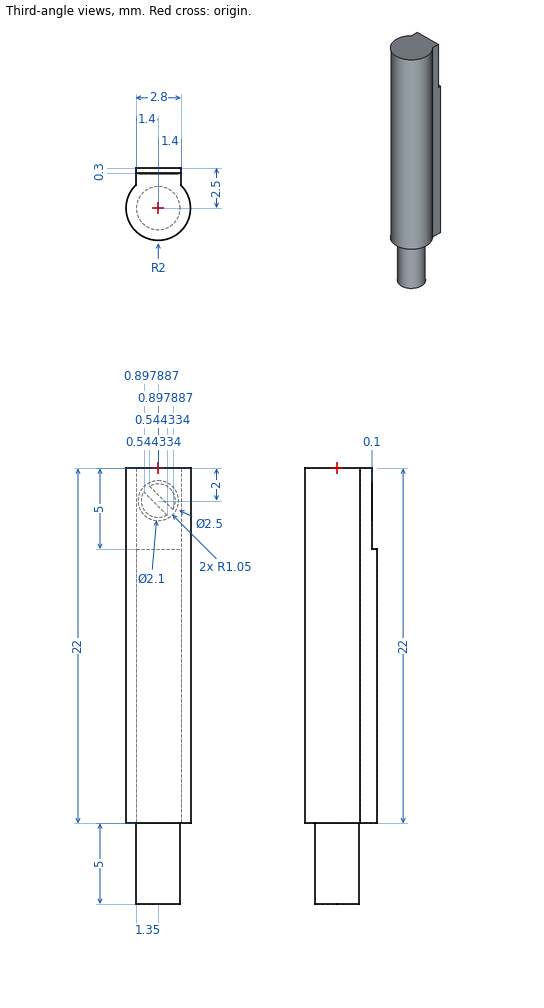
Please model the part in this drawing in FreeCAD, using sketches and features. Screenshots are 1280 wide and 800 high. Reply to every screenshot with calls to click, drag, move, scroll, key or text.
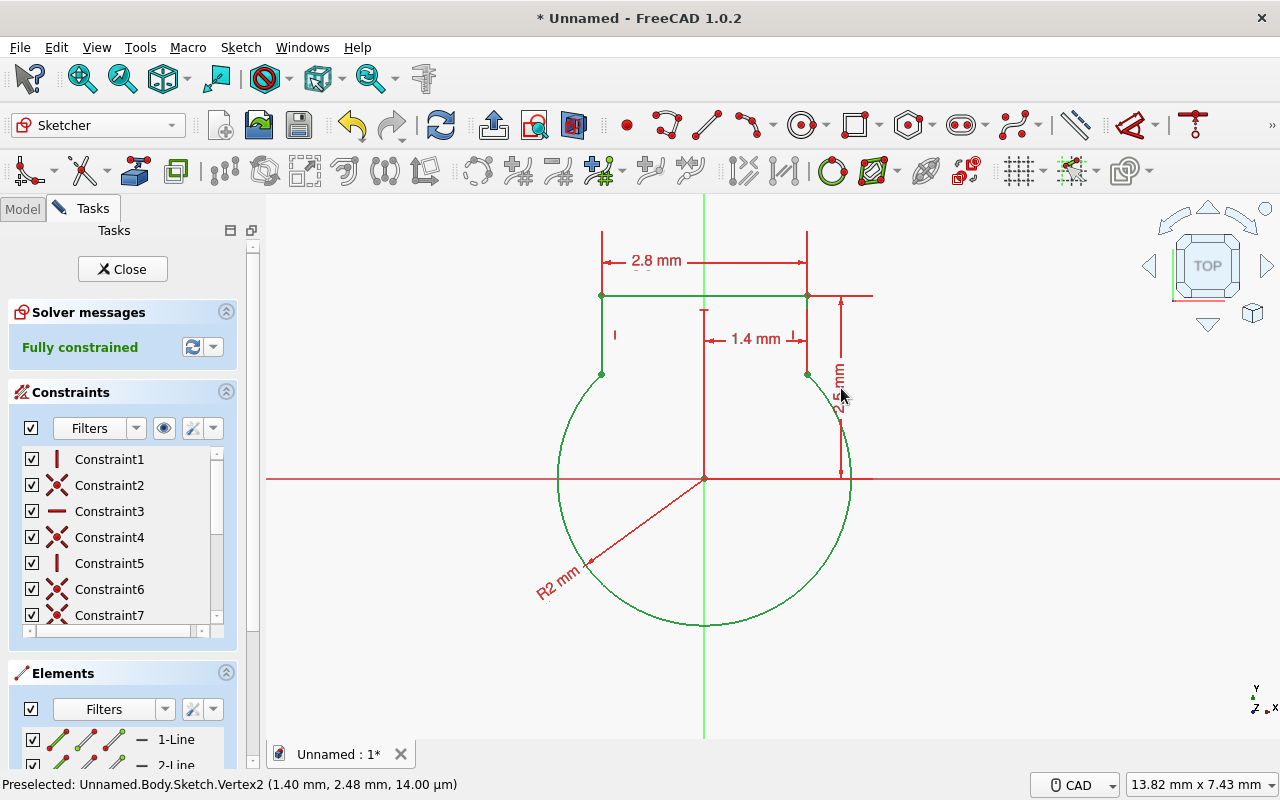
click(123, 269)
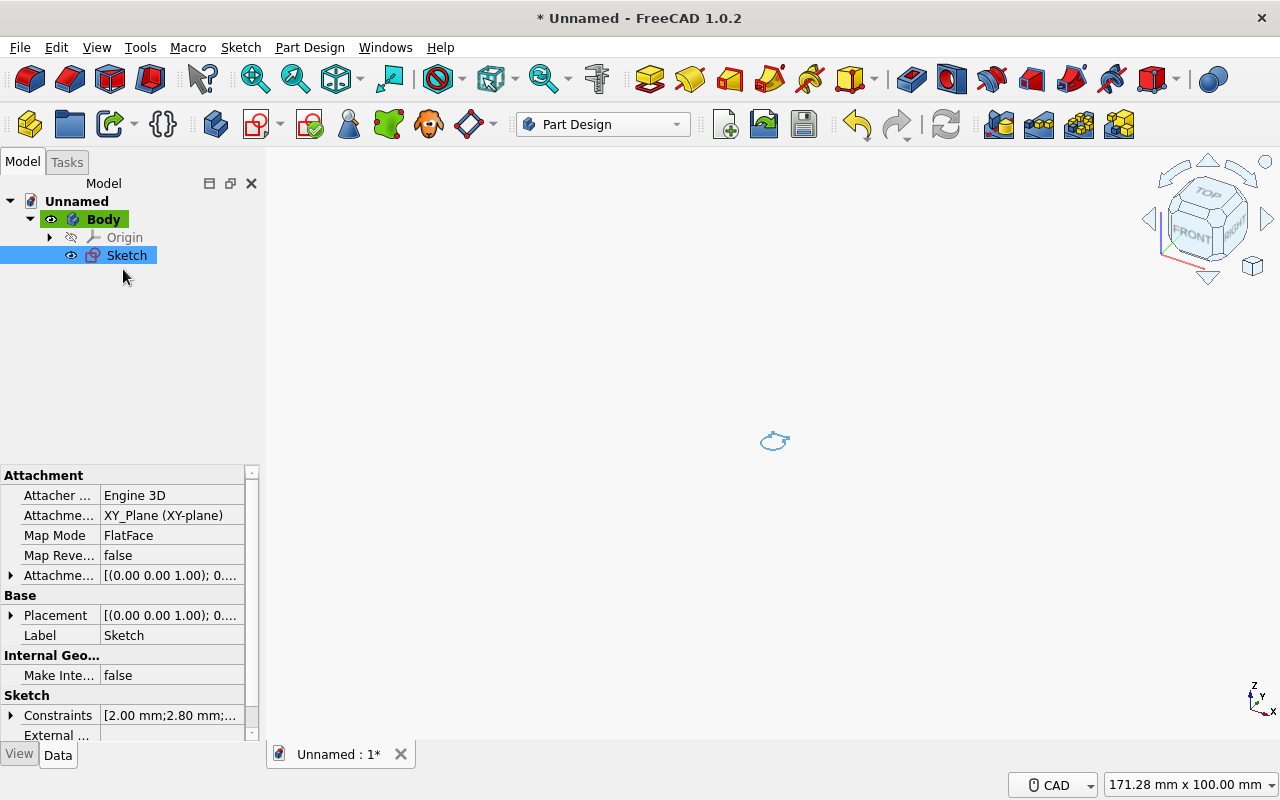
click(650, 80)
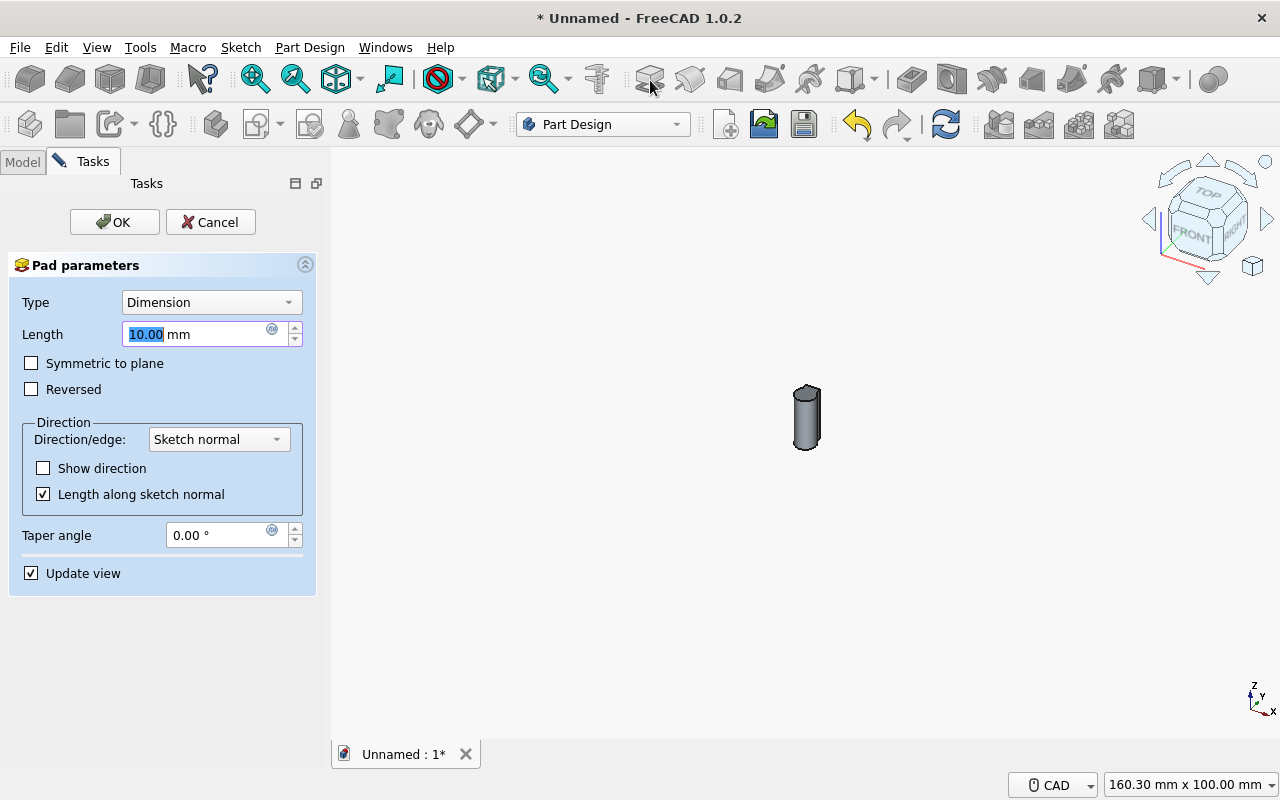
text(22)
key(Tab)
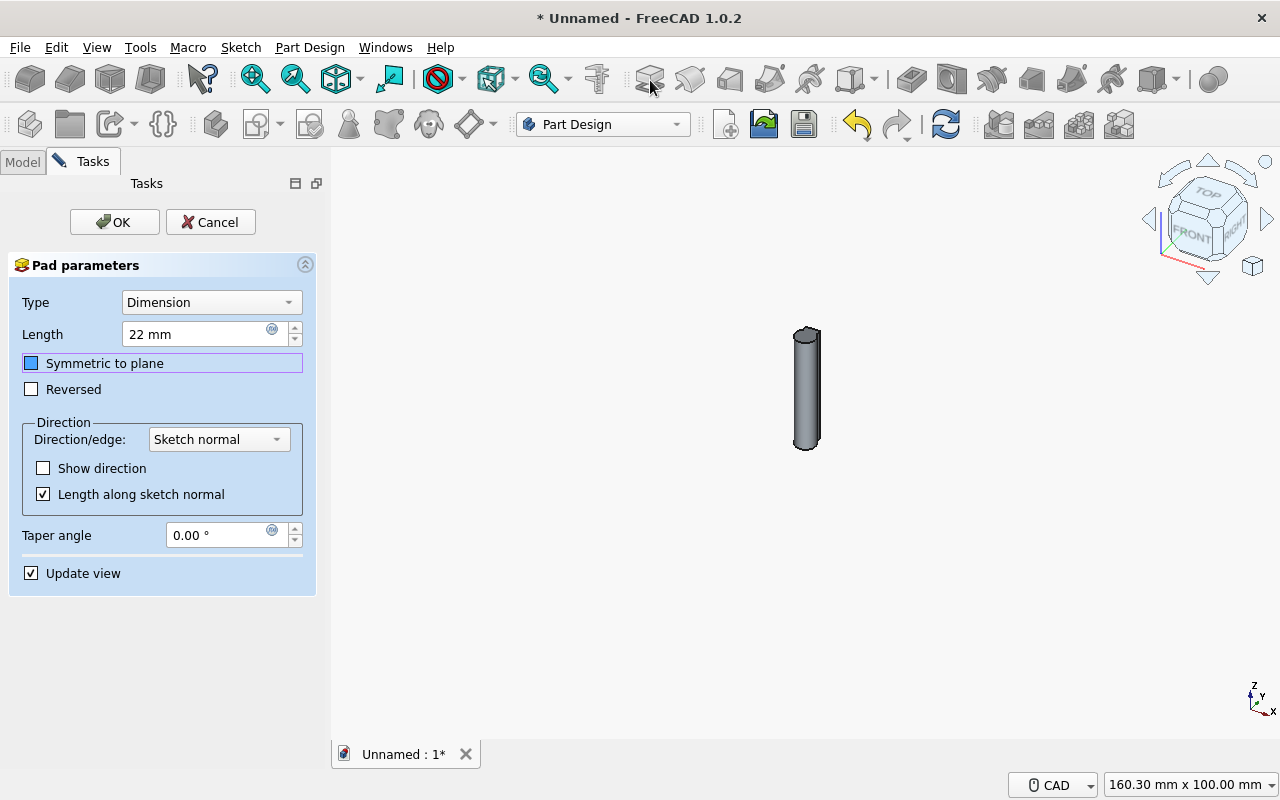
click(30, 389)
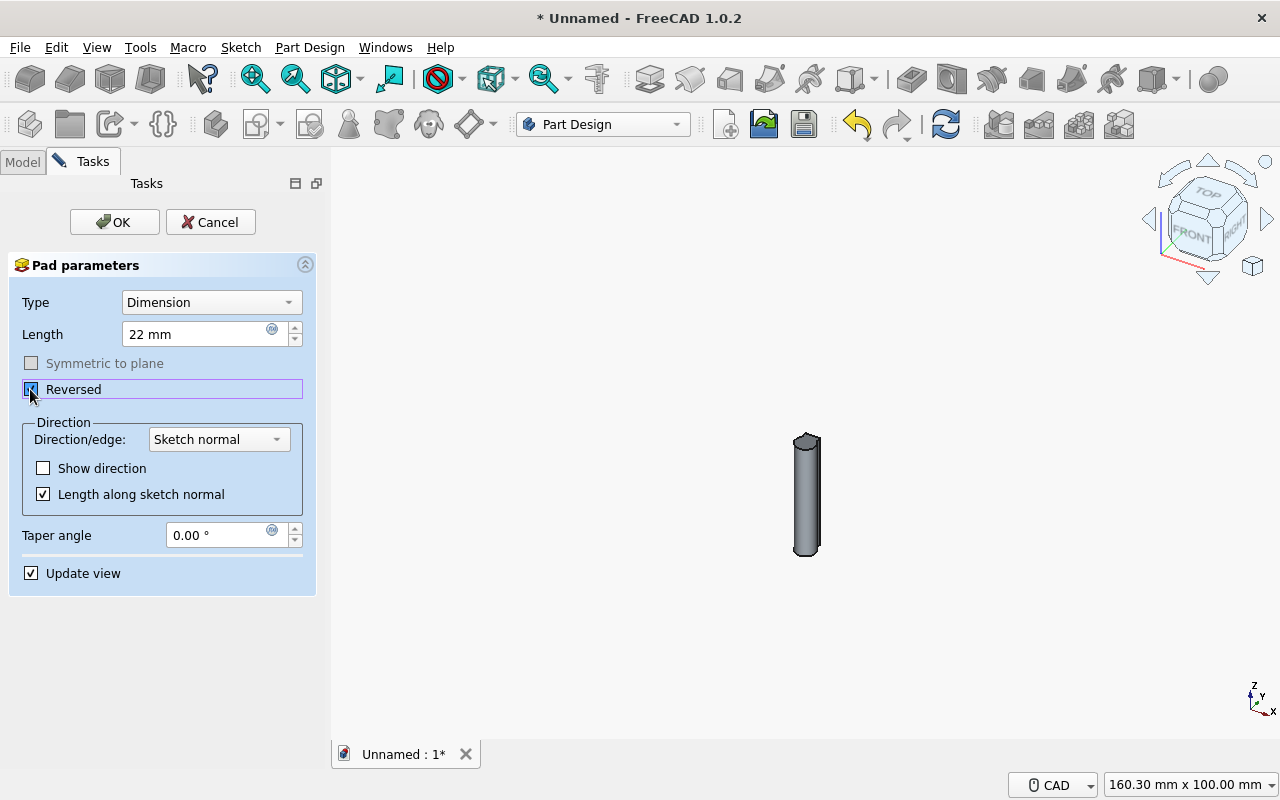
click(115, 222)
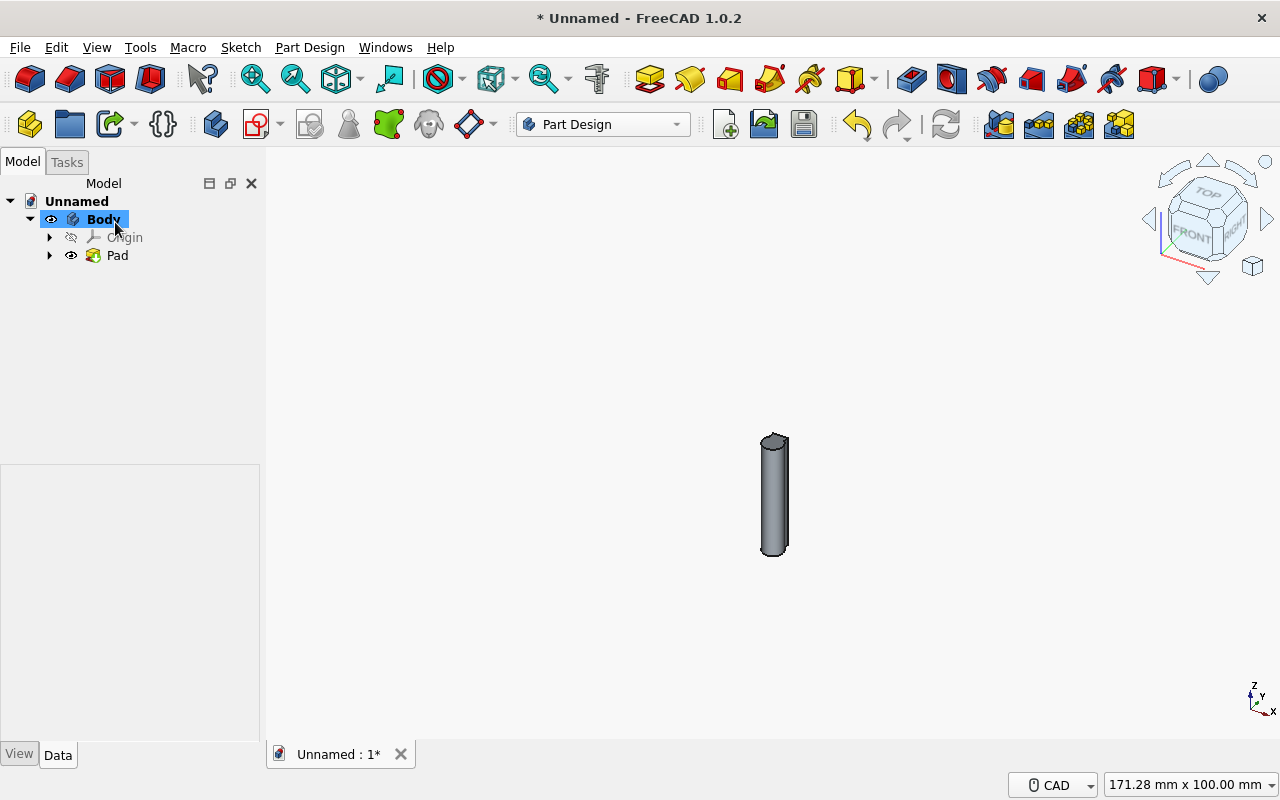
click(256, 80)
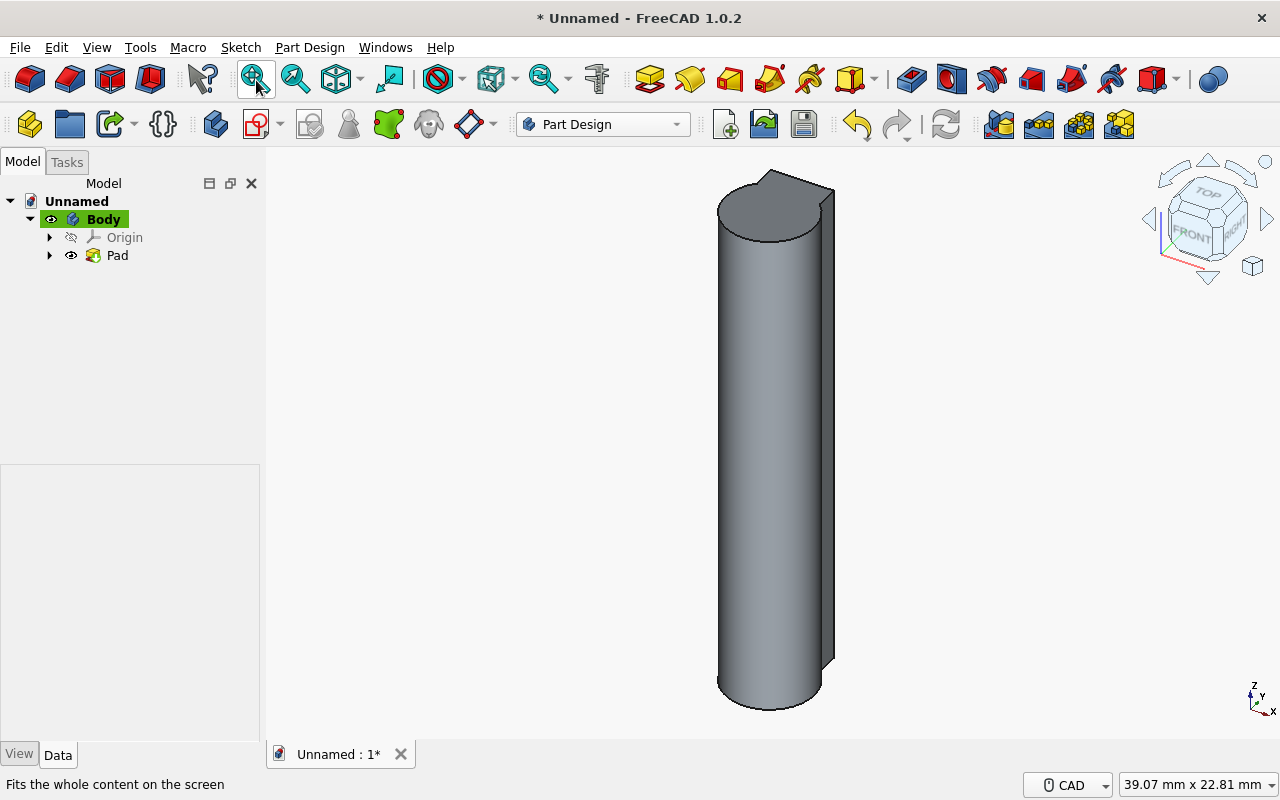
click(773, 208)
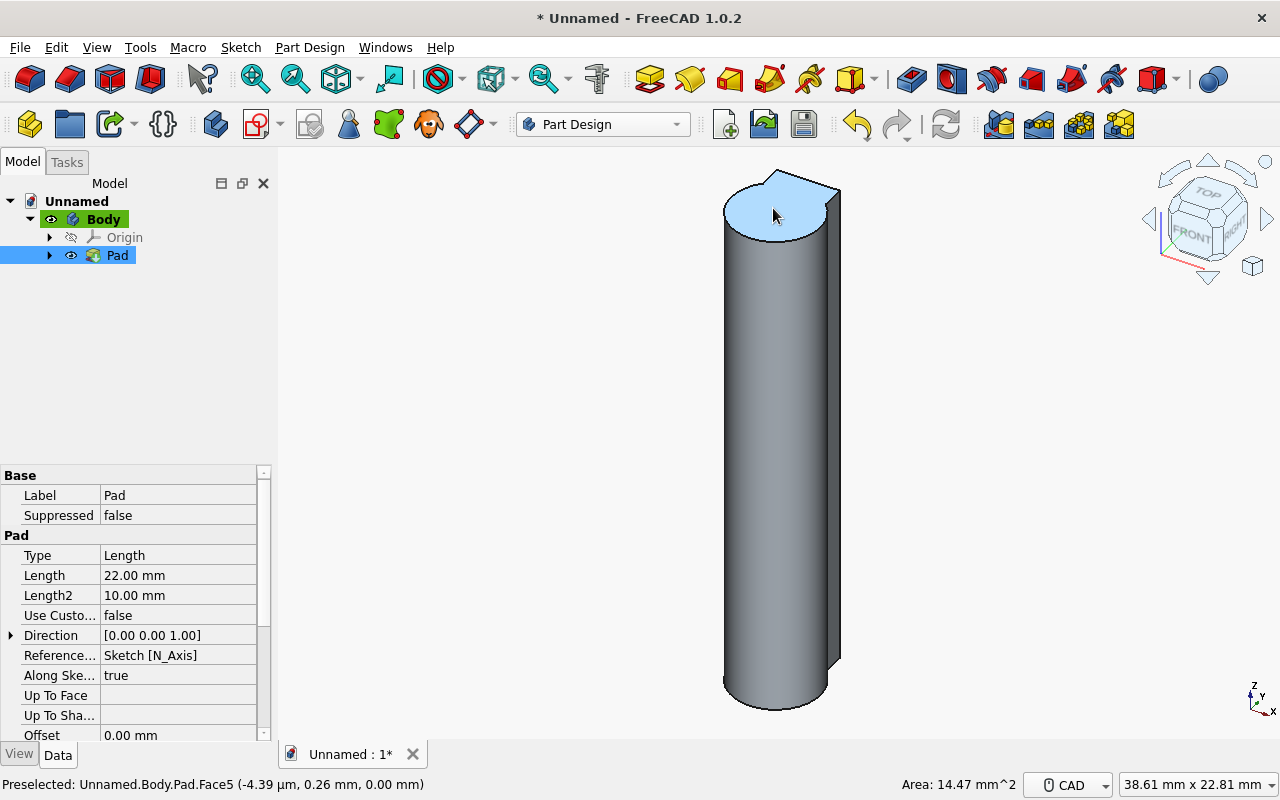
click(256, 124)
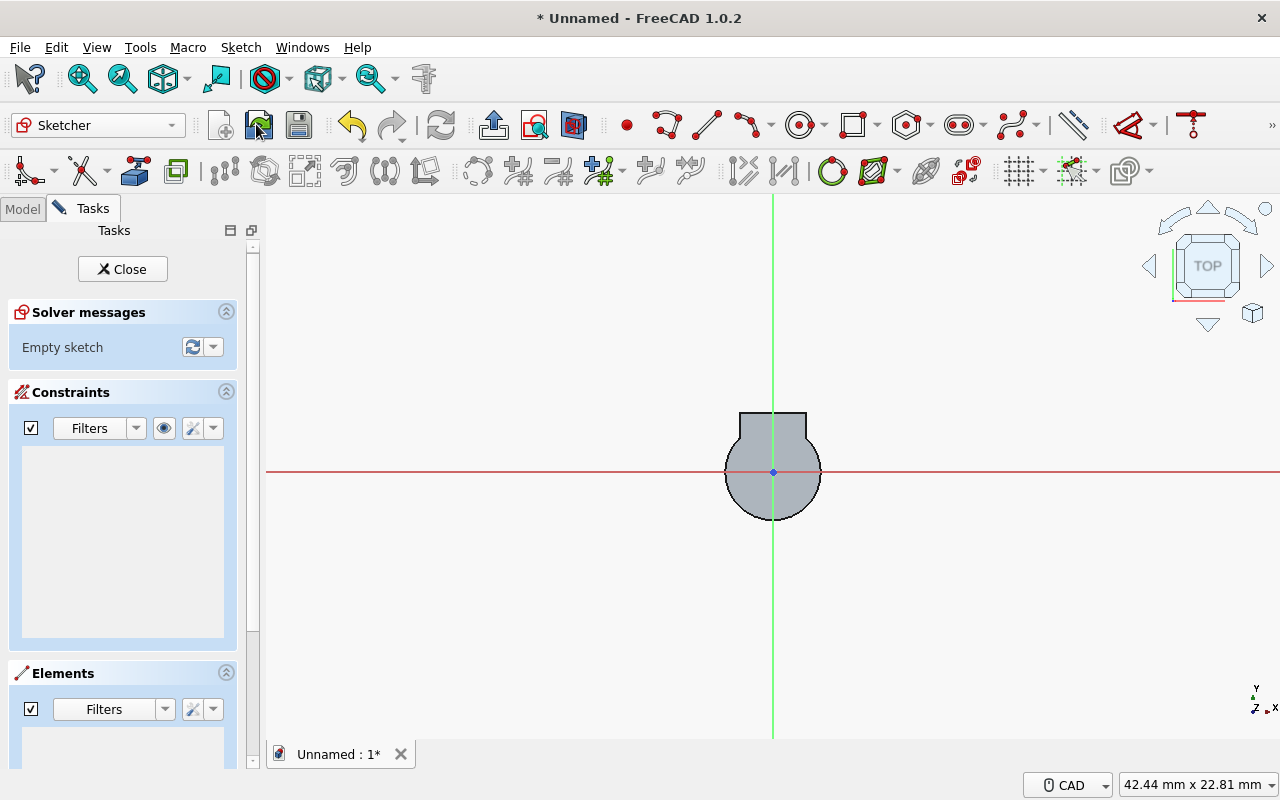
scroll(787, 438, up, 9)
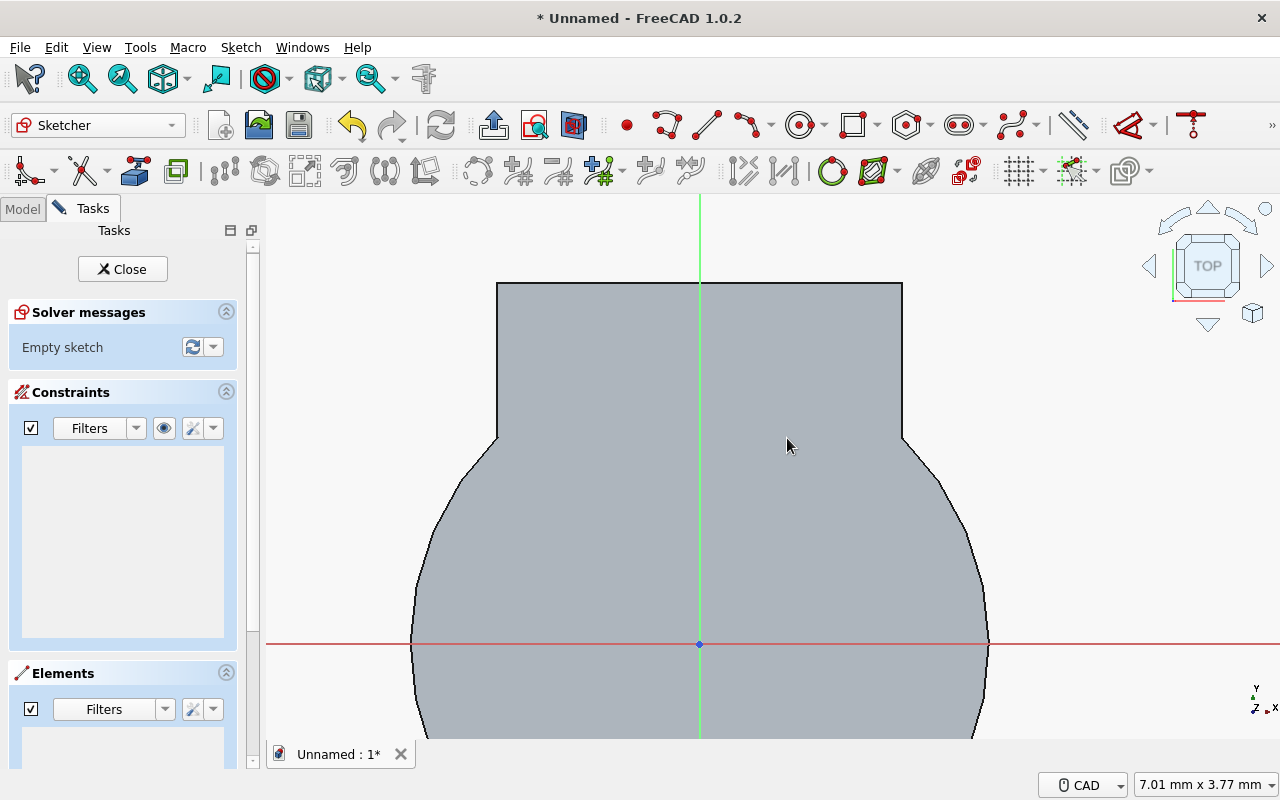
click(854, 126)